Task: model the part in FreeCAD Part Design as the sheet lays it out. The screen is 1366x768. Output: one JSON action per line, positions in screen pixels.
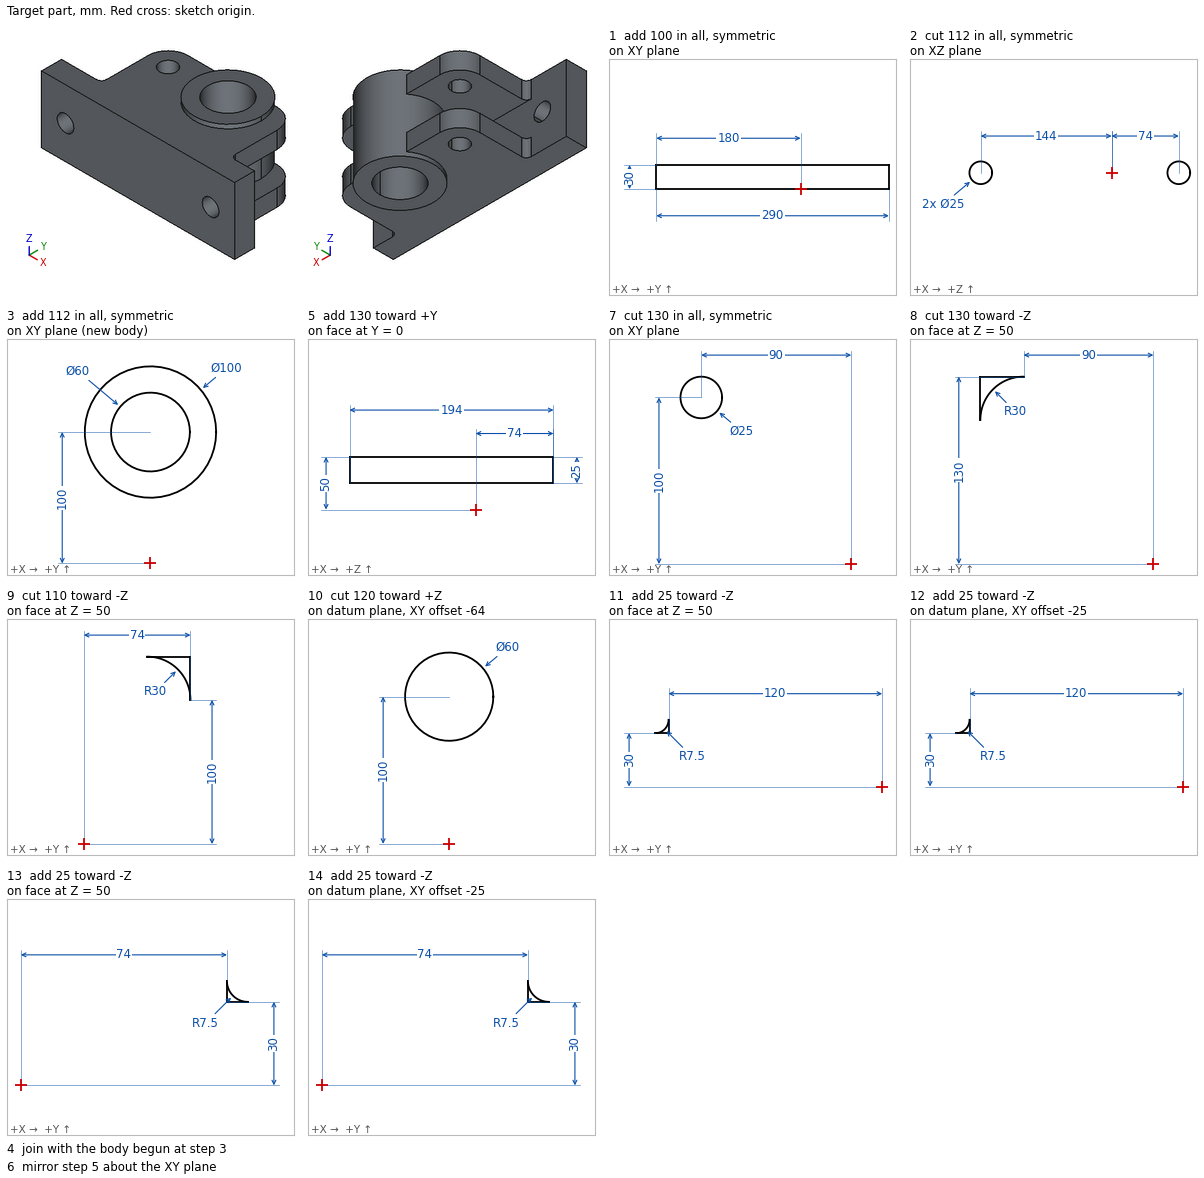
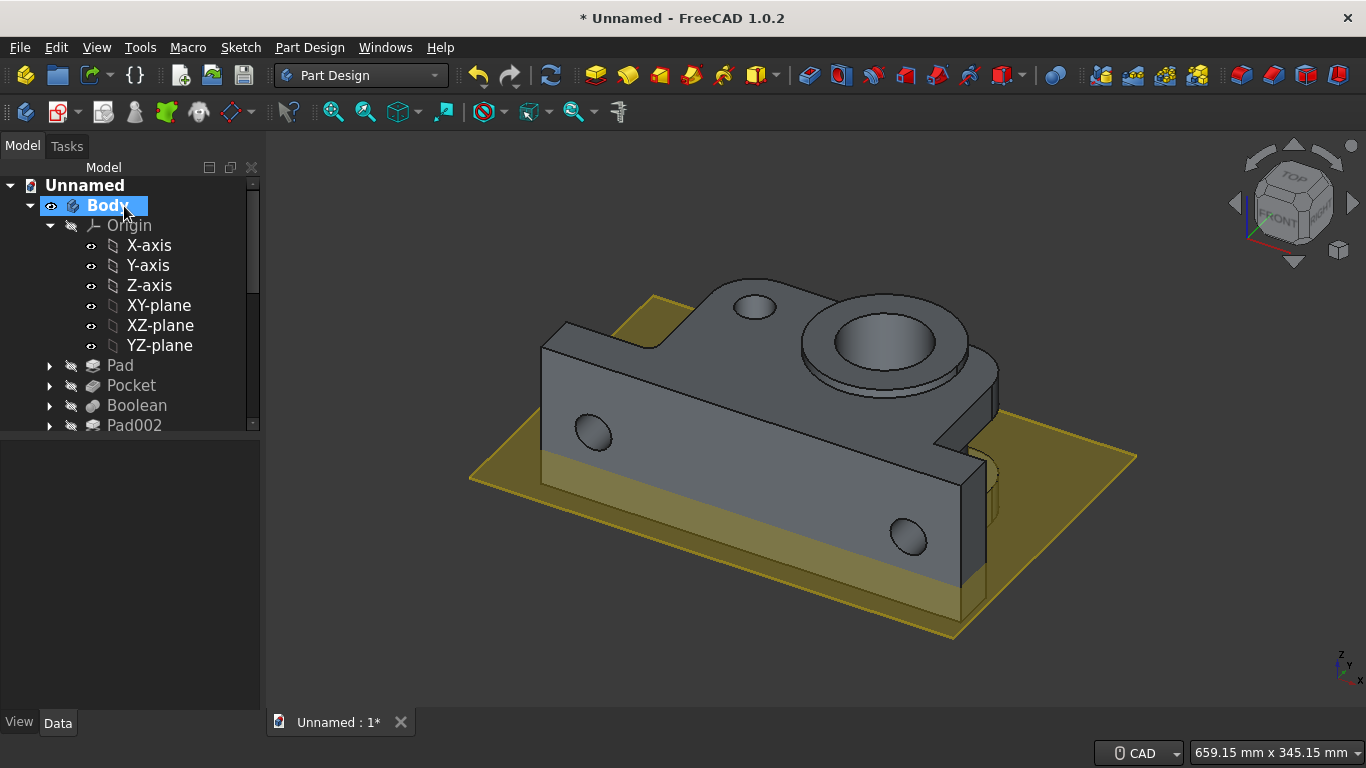
{"action": "scroll", "coordinate": [100, 301], "scroll_direction": "down", "scroll_amount": 3}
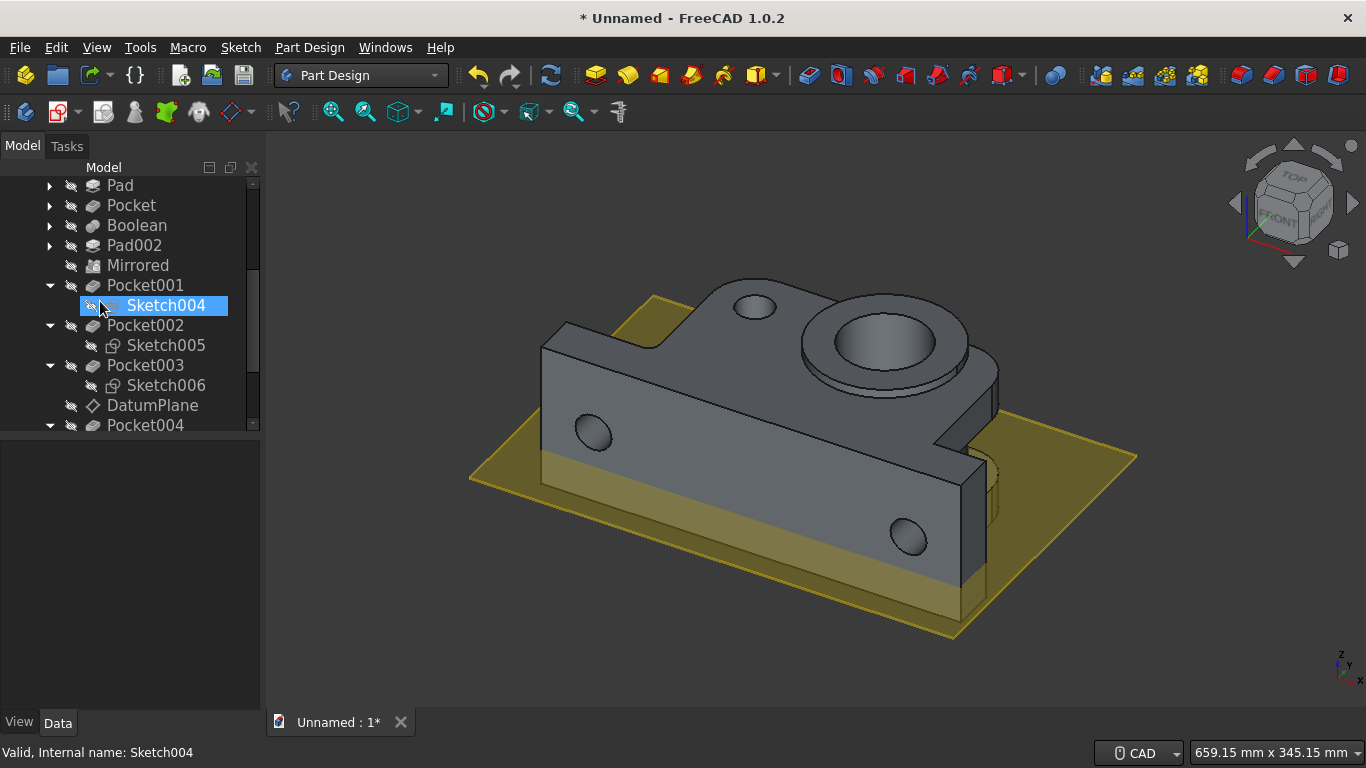
{"action": "scroll", "coordinate": [140, 301], "scroll_direction": "up", "scroll_amount": 15}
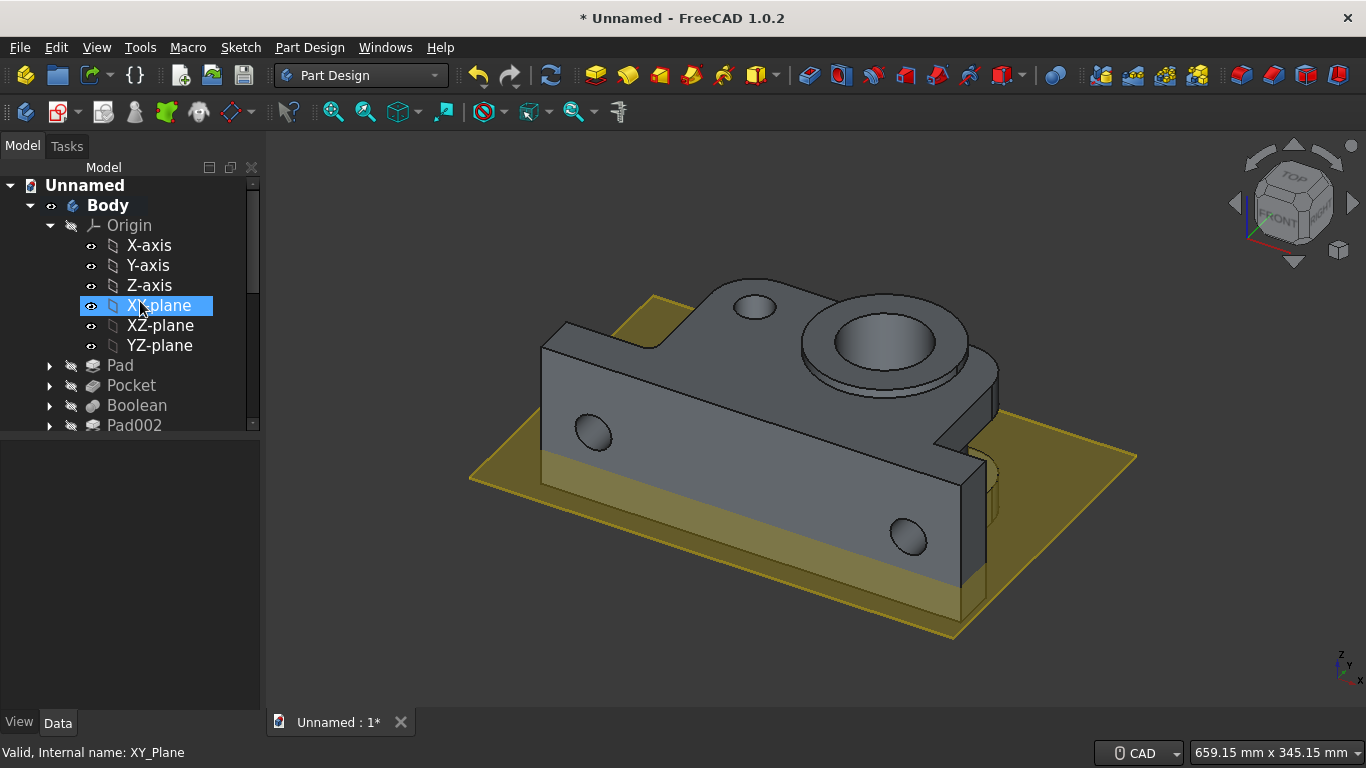
{"action": "scroll", "coordinate": [100, 301], "scroll_direction": "down", "scroll_amount": 6}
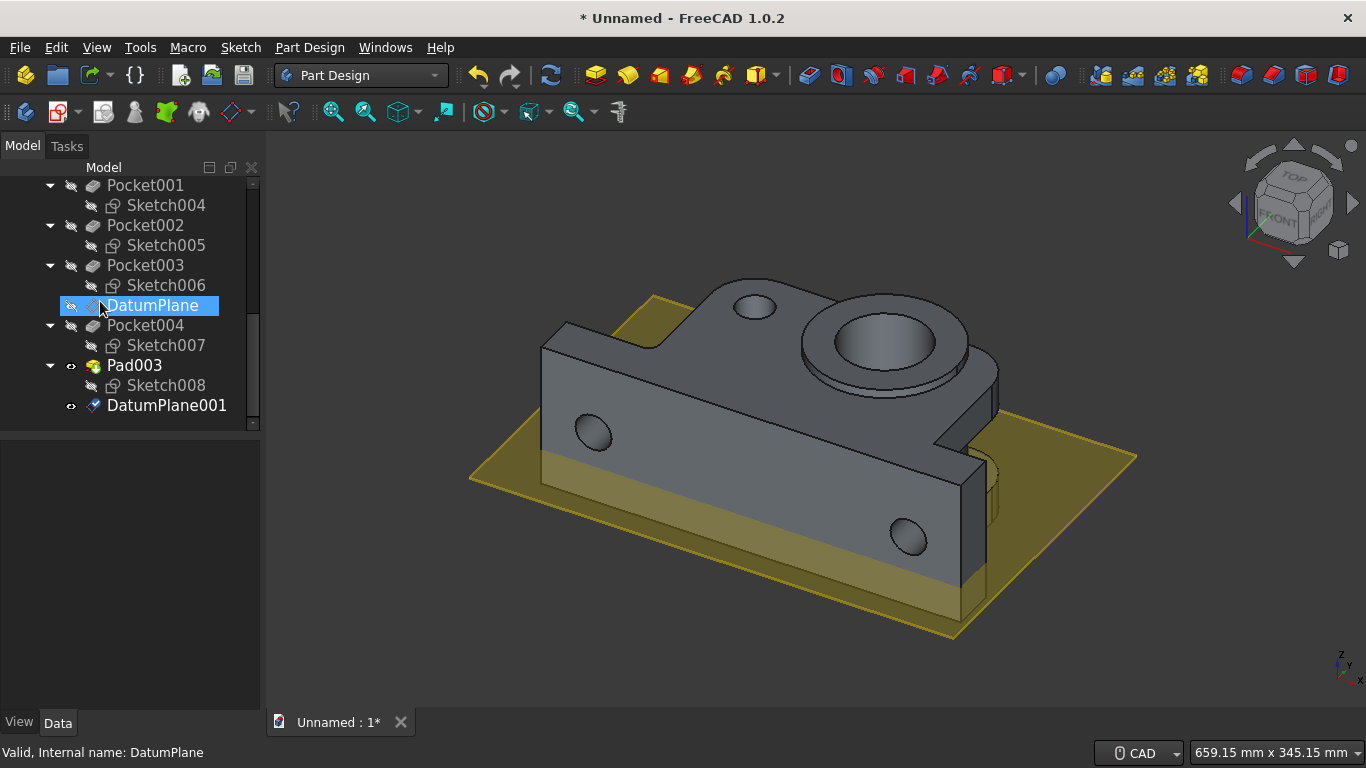
{"action": "left_click", "coordinate": [116, 406]}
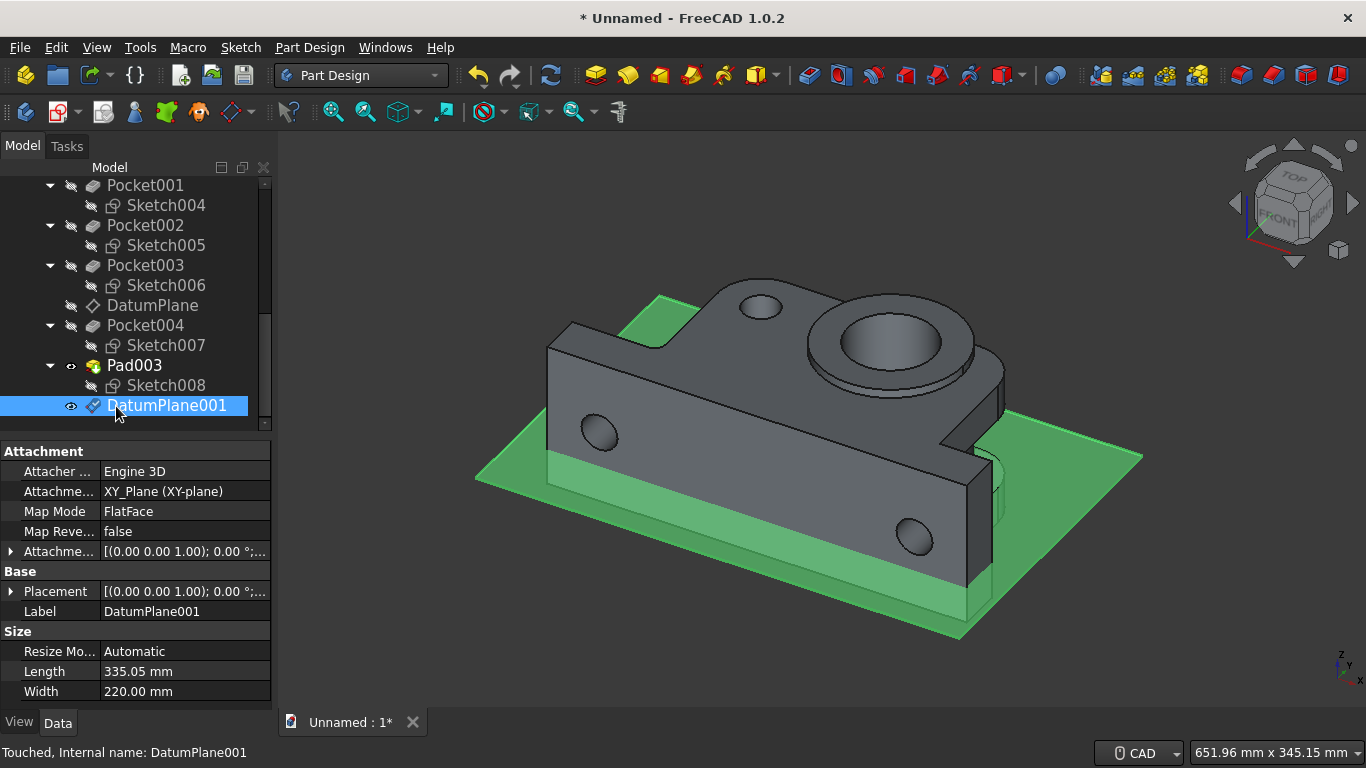
{"action": "left_click", "coordinate": [58, 112]}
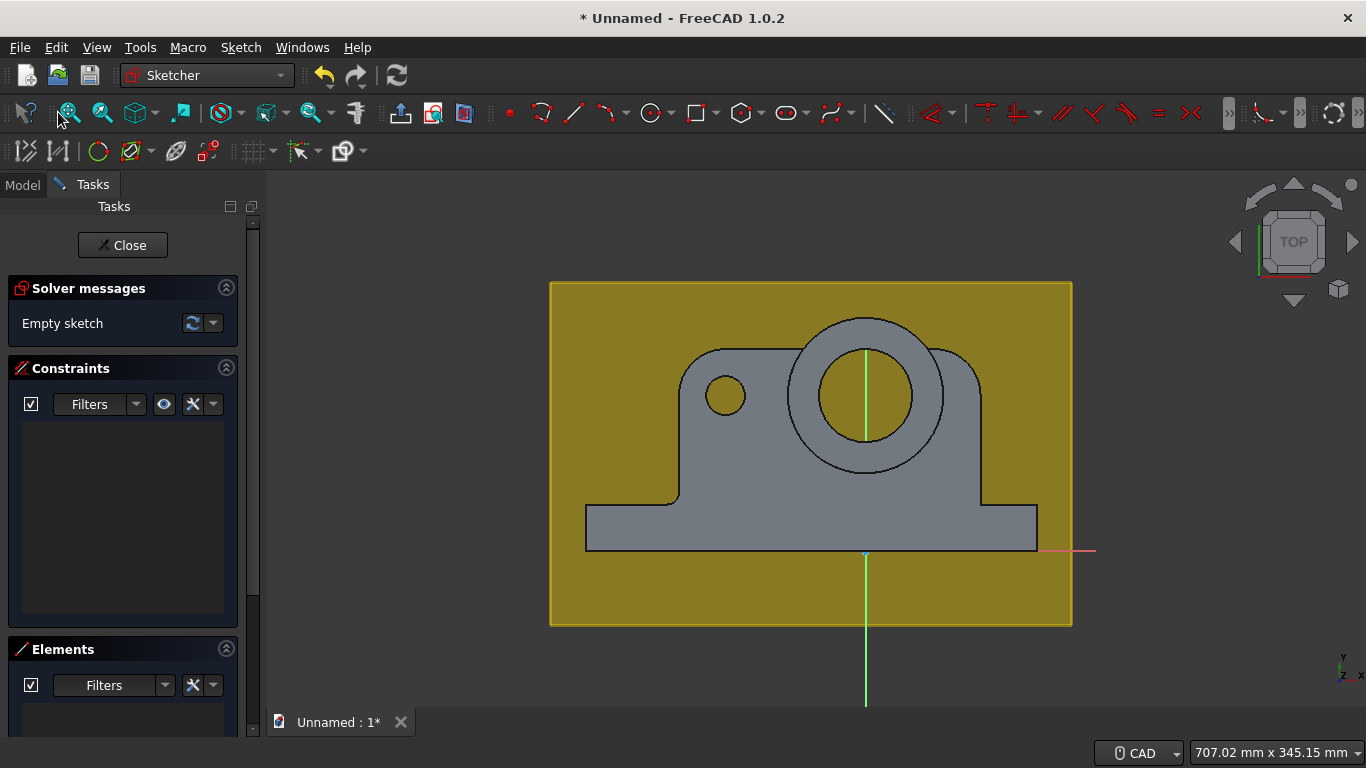
{"action": "left_click", "coordinate": [466, 114]}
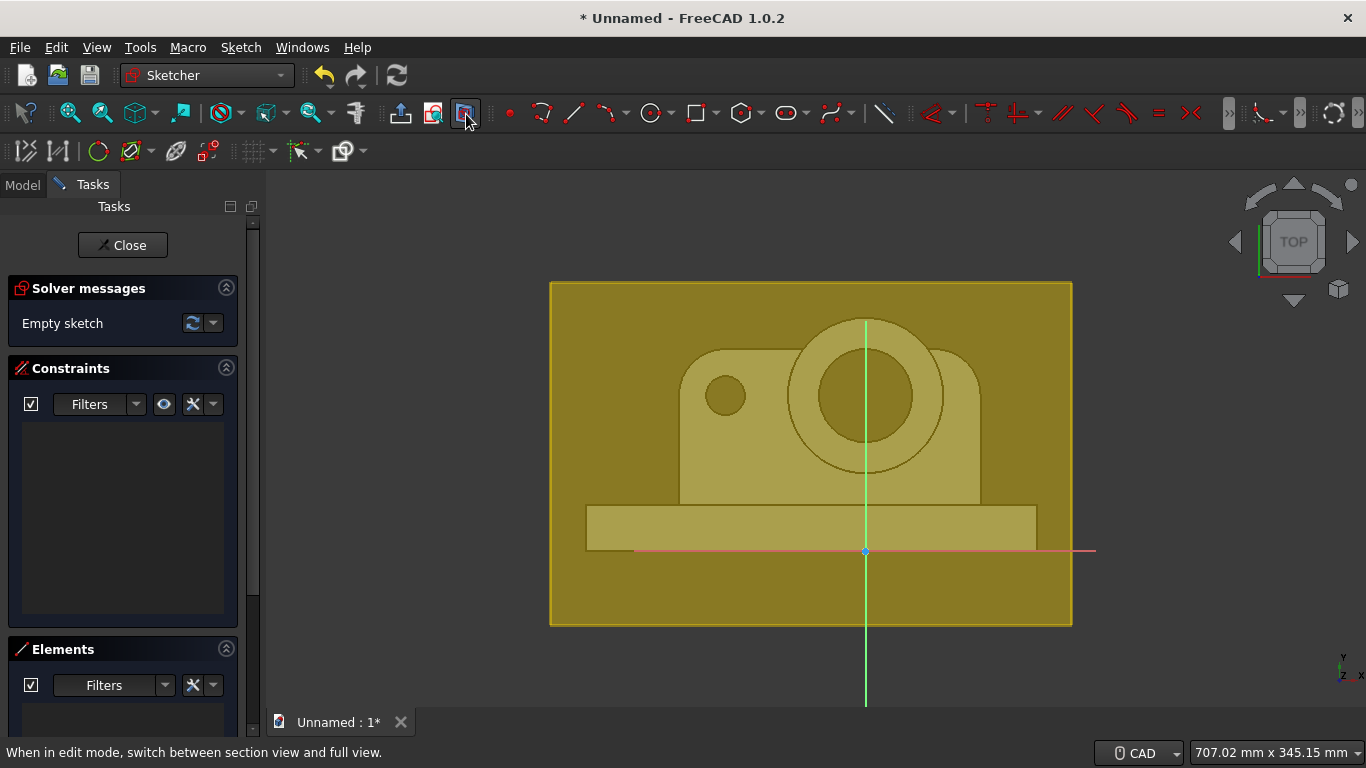
{"action": "scroll", "coordinate": [669, 502], "scroll_direction": "up", "scroll_amount": 15}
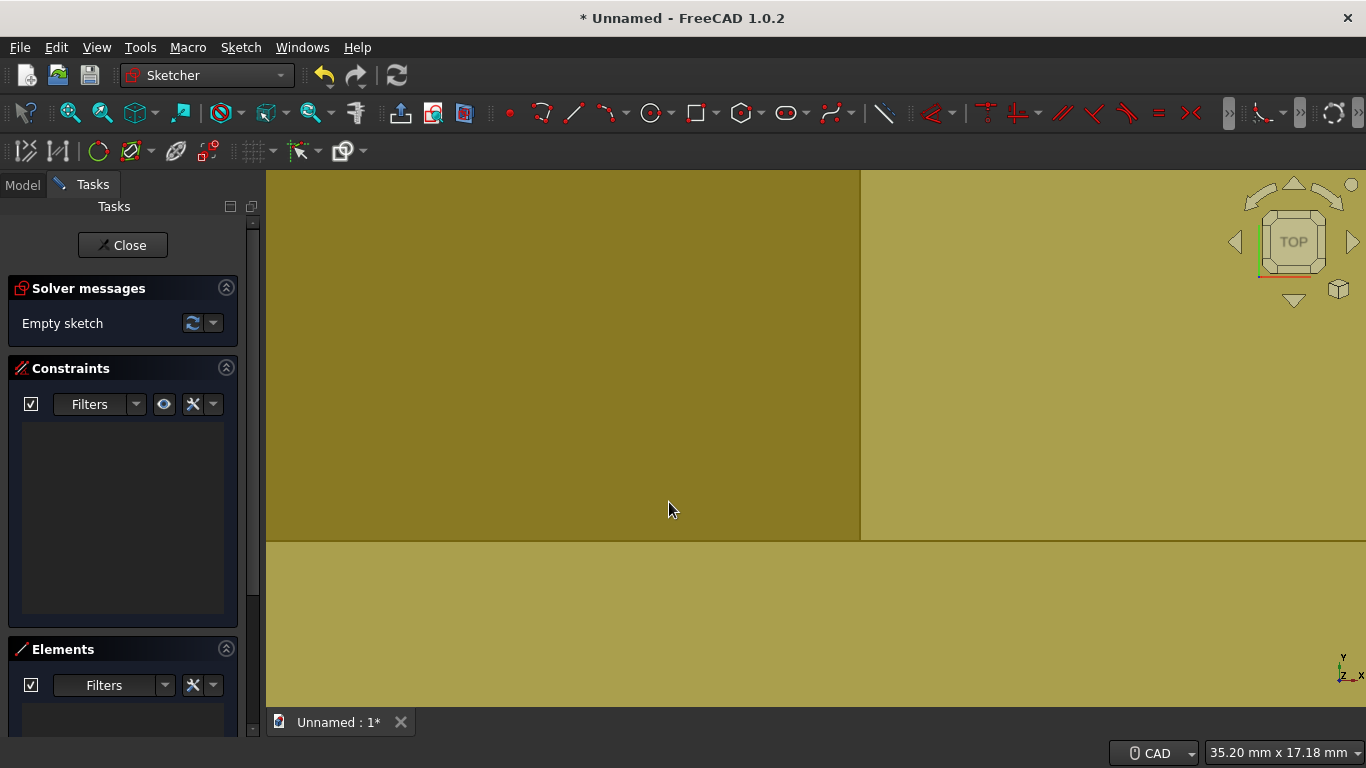
{"action": "scroll", "coordinate": [734, 393], "scroll_direction": "up", "scroll_amount": 2}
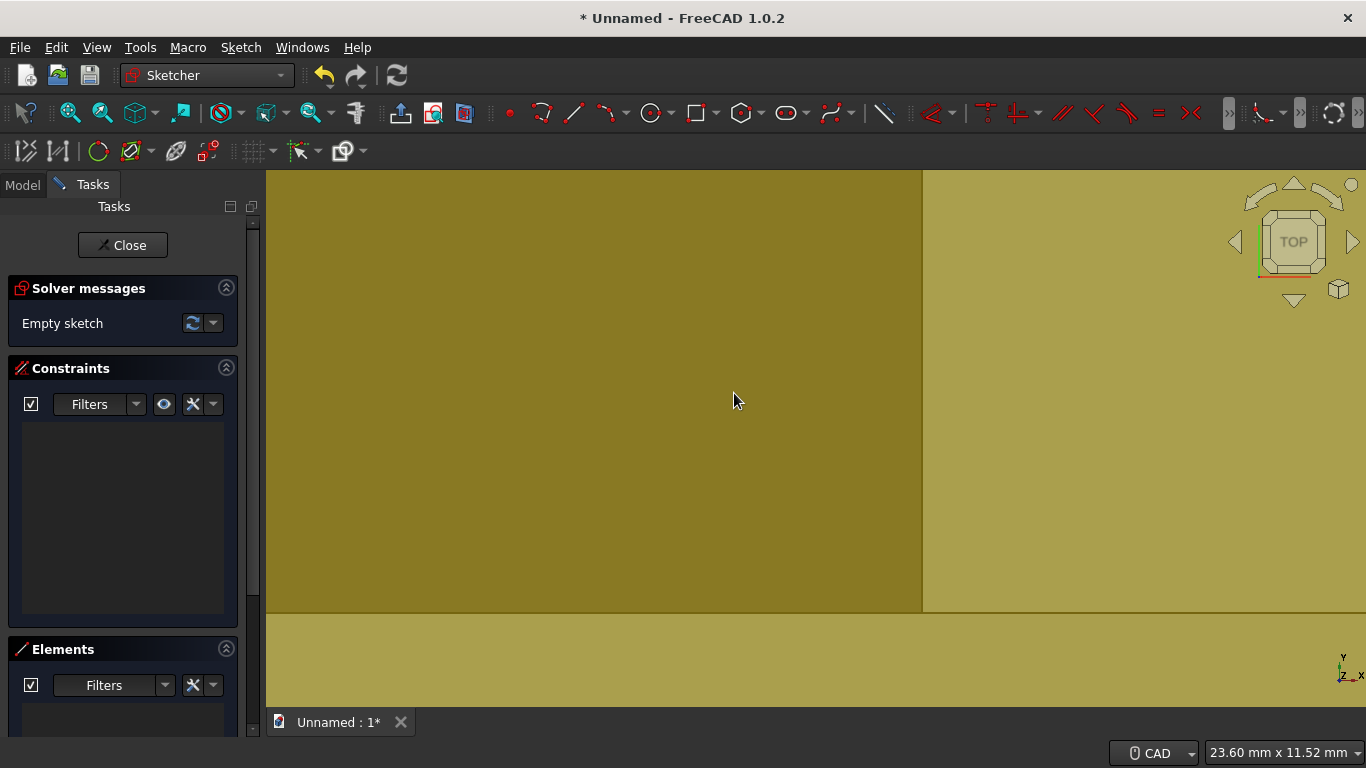
{"action": "left_click", "coordinate": [542, 114]}